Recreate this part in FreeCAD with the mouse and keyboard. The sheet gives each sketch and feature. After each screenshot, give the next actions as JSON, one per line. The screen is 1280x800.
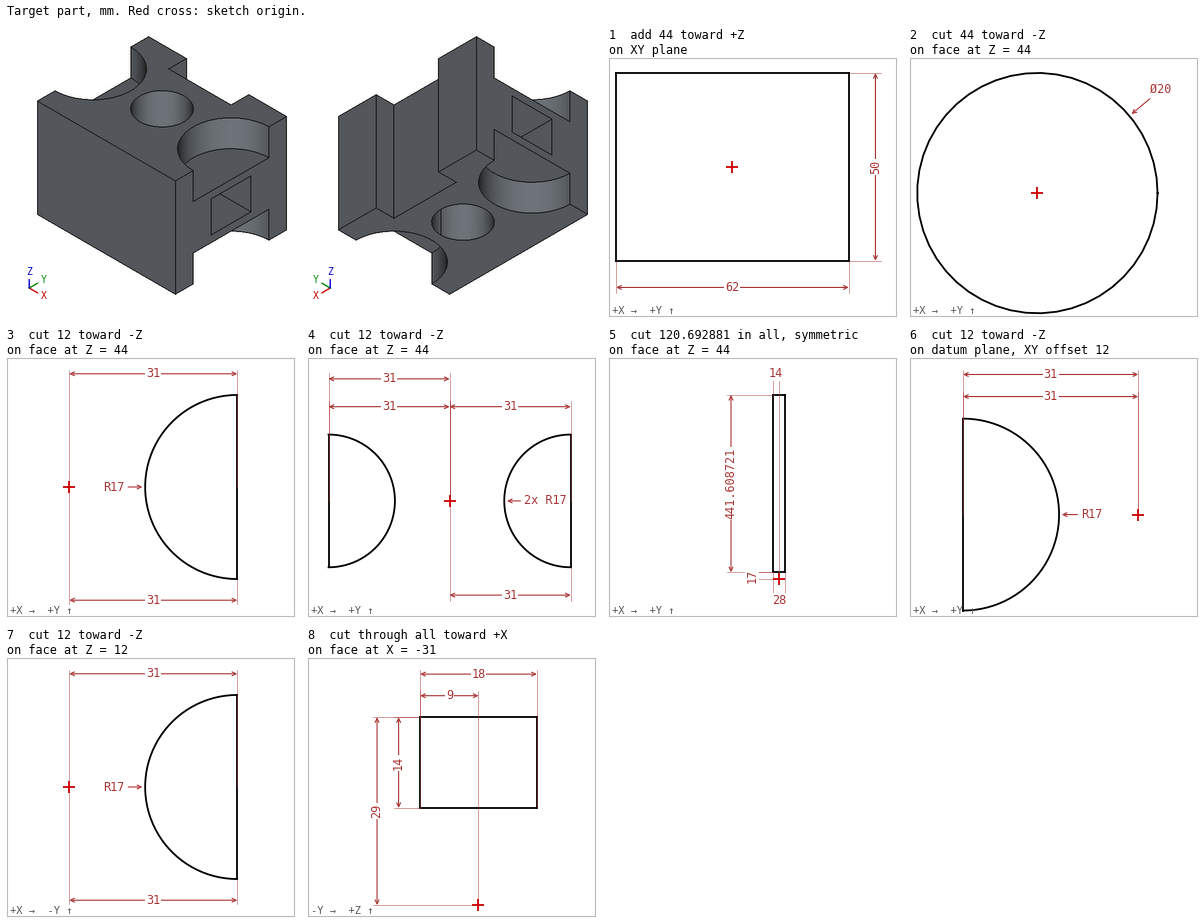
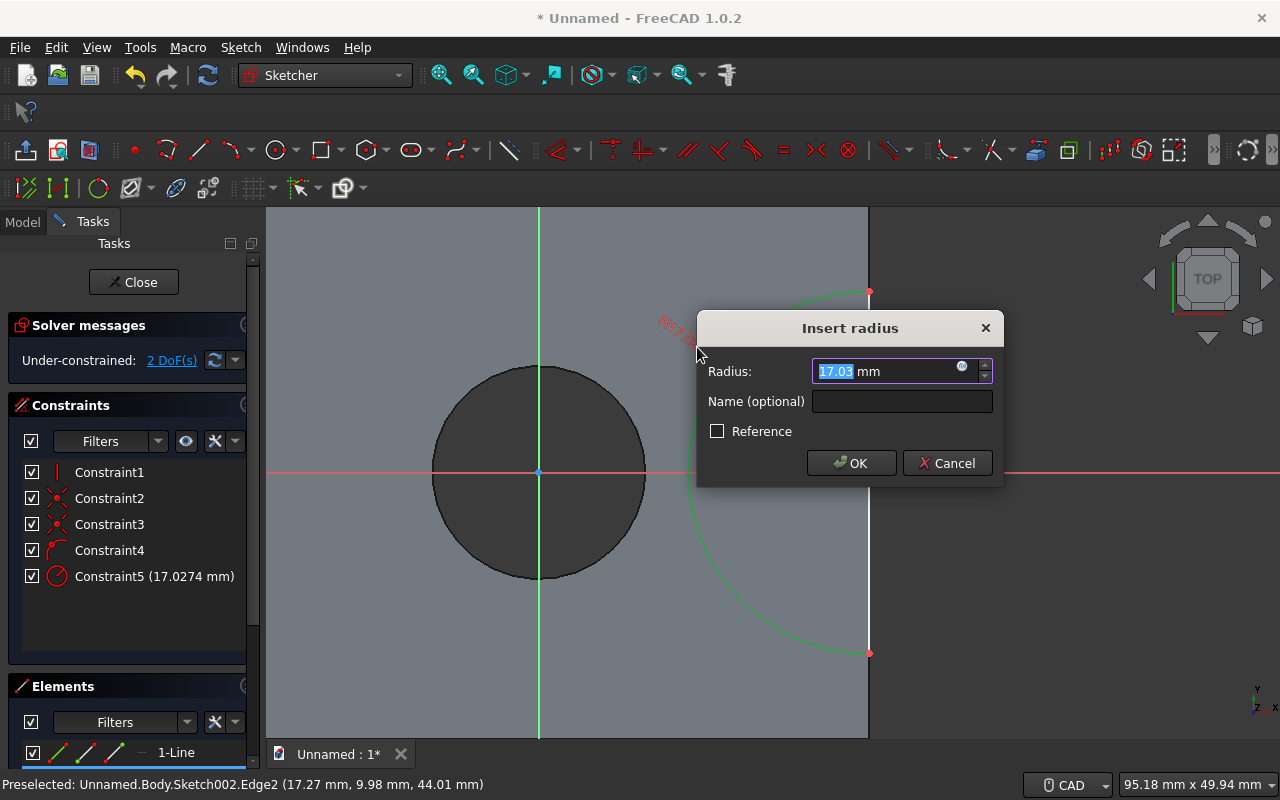
{"action": "type", "text": "17"}
{"action": "key", "text": "Return"}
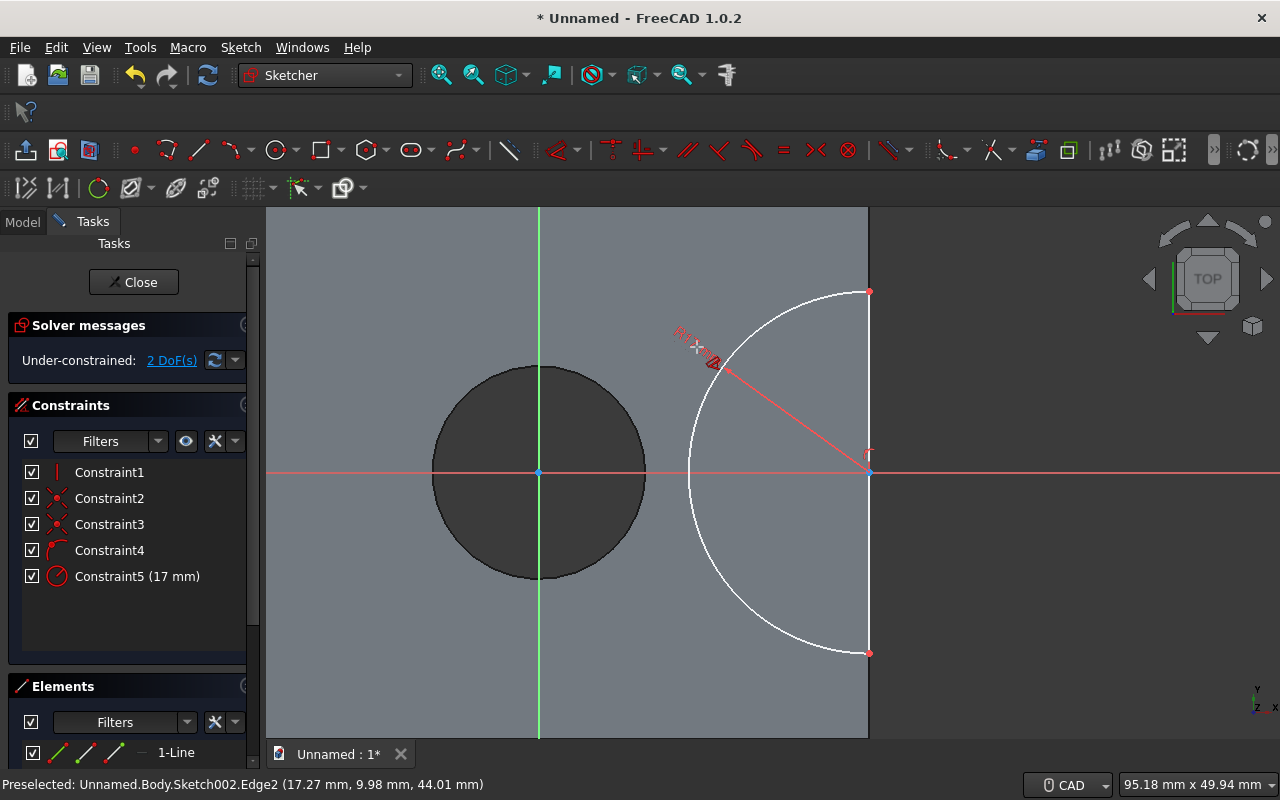
{"action": "left_click", "coordinate": [869, 654]}
{"action": "left_click", "coordinate": [704, 688]}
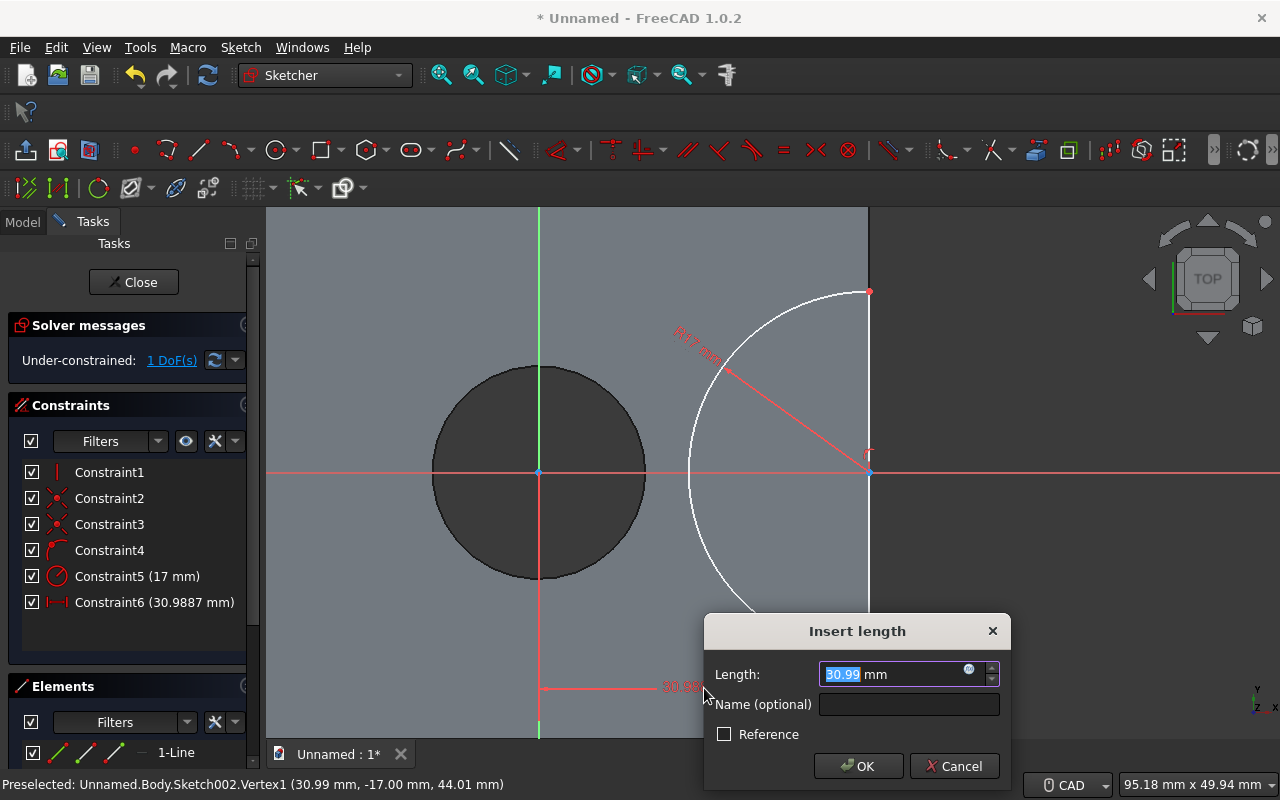
{"action": "type", "text": "31"}
{"action": "key", "text": "Return"}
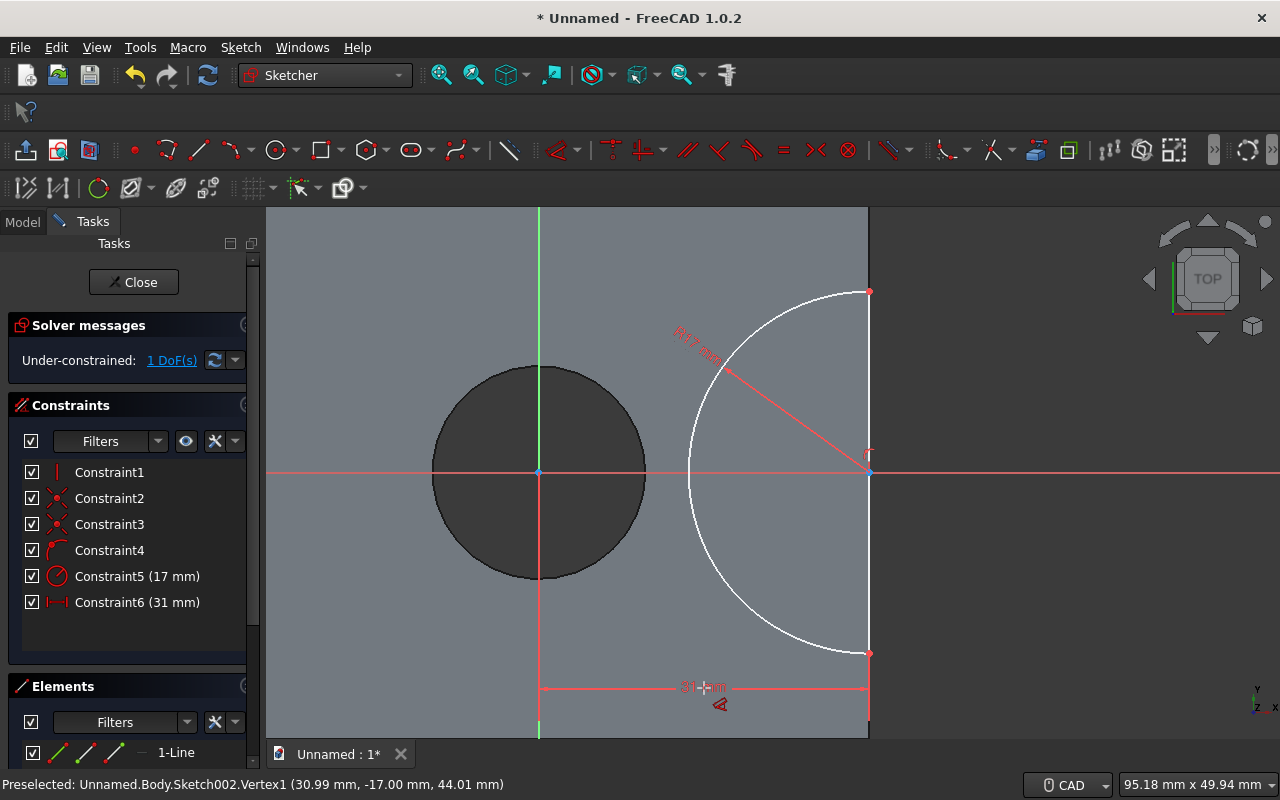
{"action": "left_click", "coordinate": [870, 473]}
{"action": "left_click", "coordinate": [628, 507]}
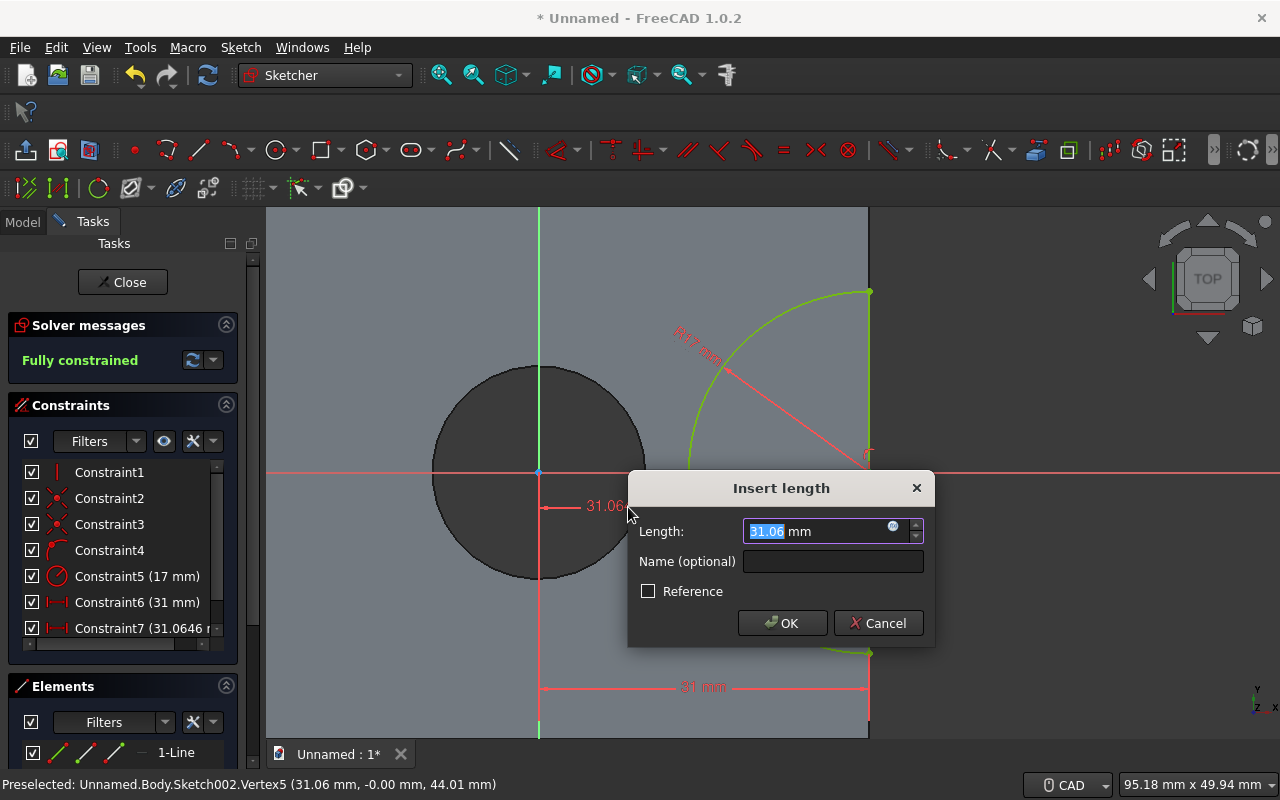
{"action": "type", "text": "31"}
{"action": "key", "text": "Return"}
{"action": "key", "text": "Escape"}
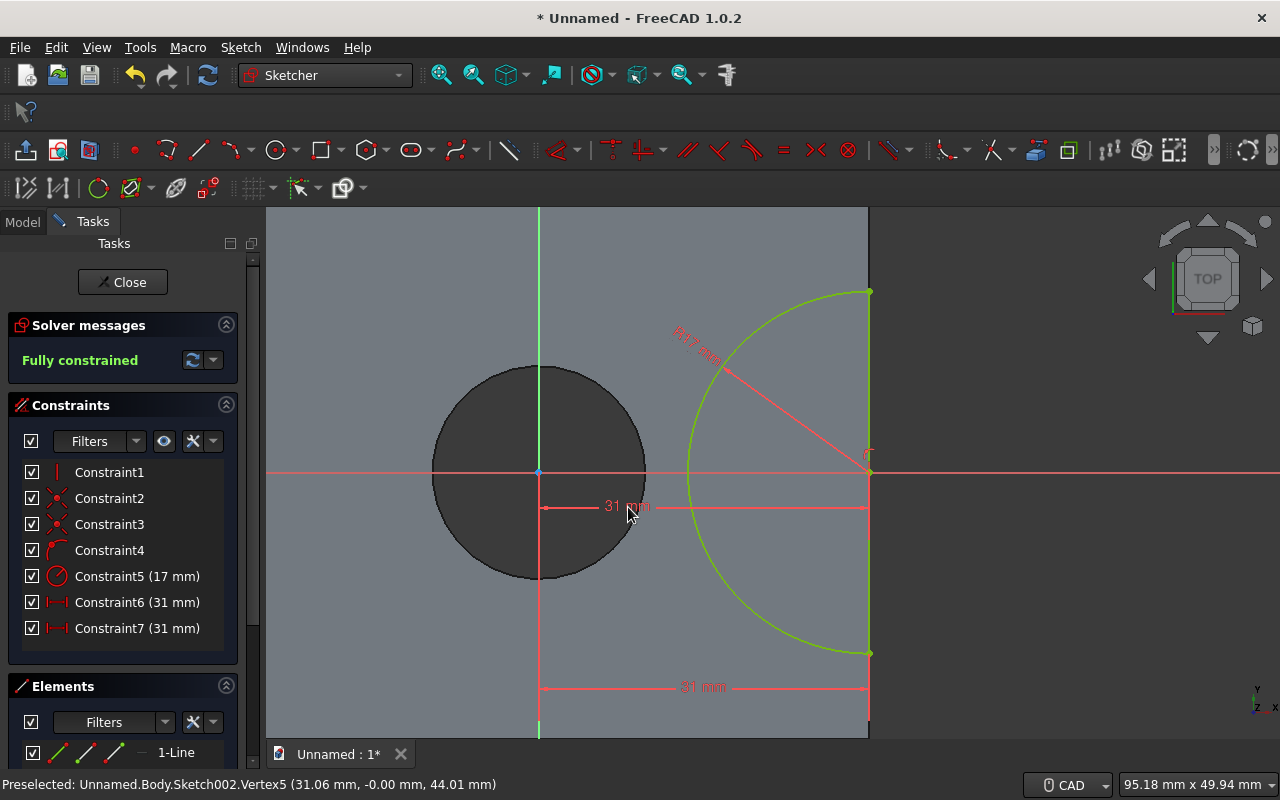
{"action": "left_click", "coordinate": [123, 282]}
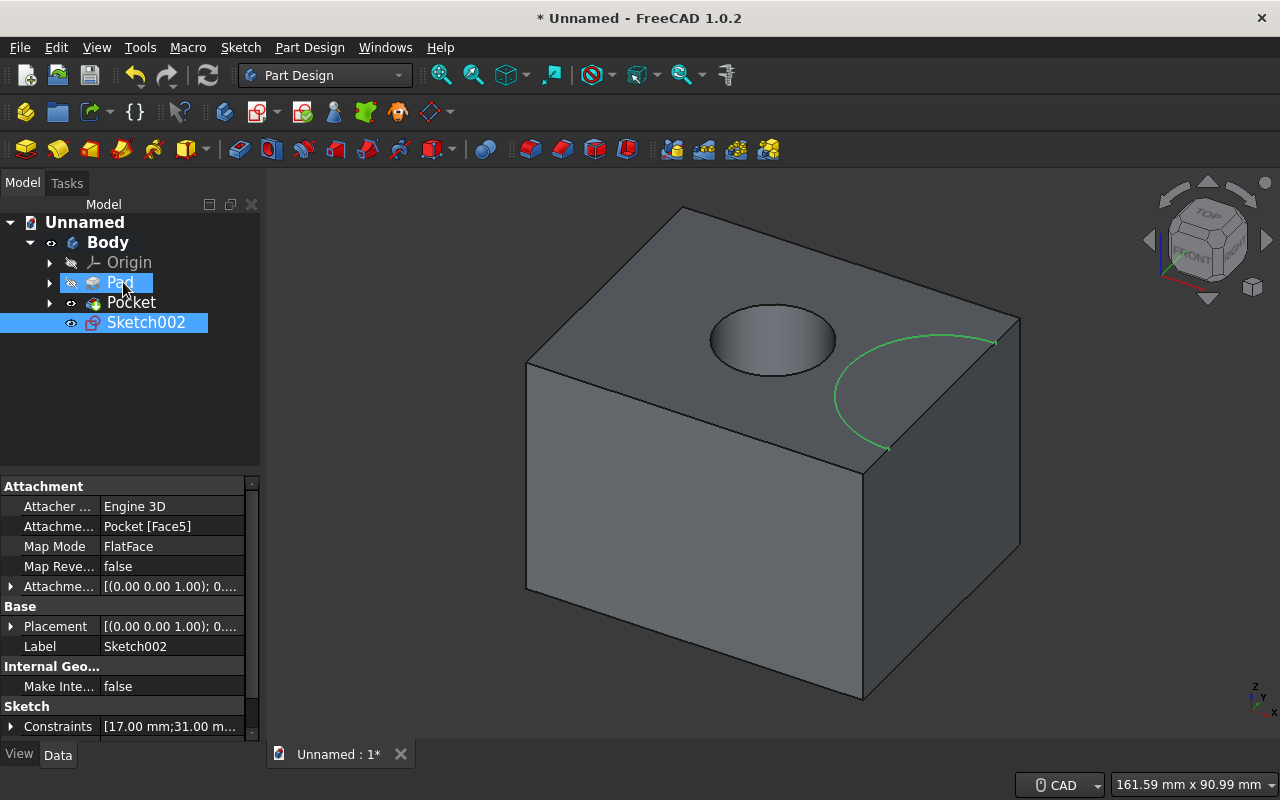
{"action": "left_click", "coordinate": [240, 150]}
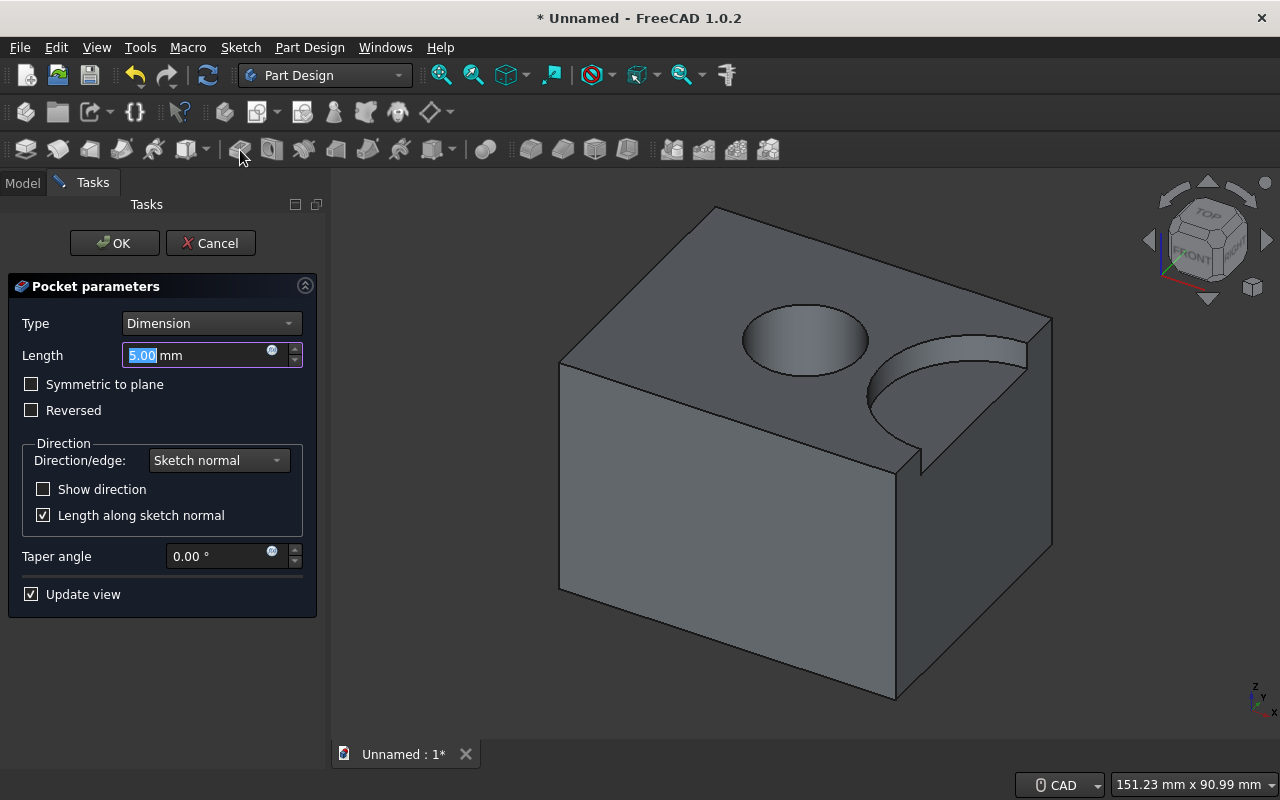
{"action": "type", "text": "12"}
{"action": "key", "text": "Tab"}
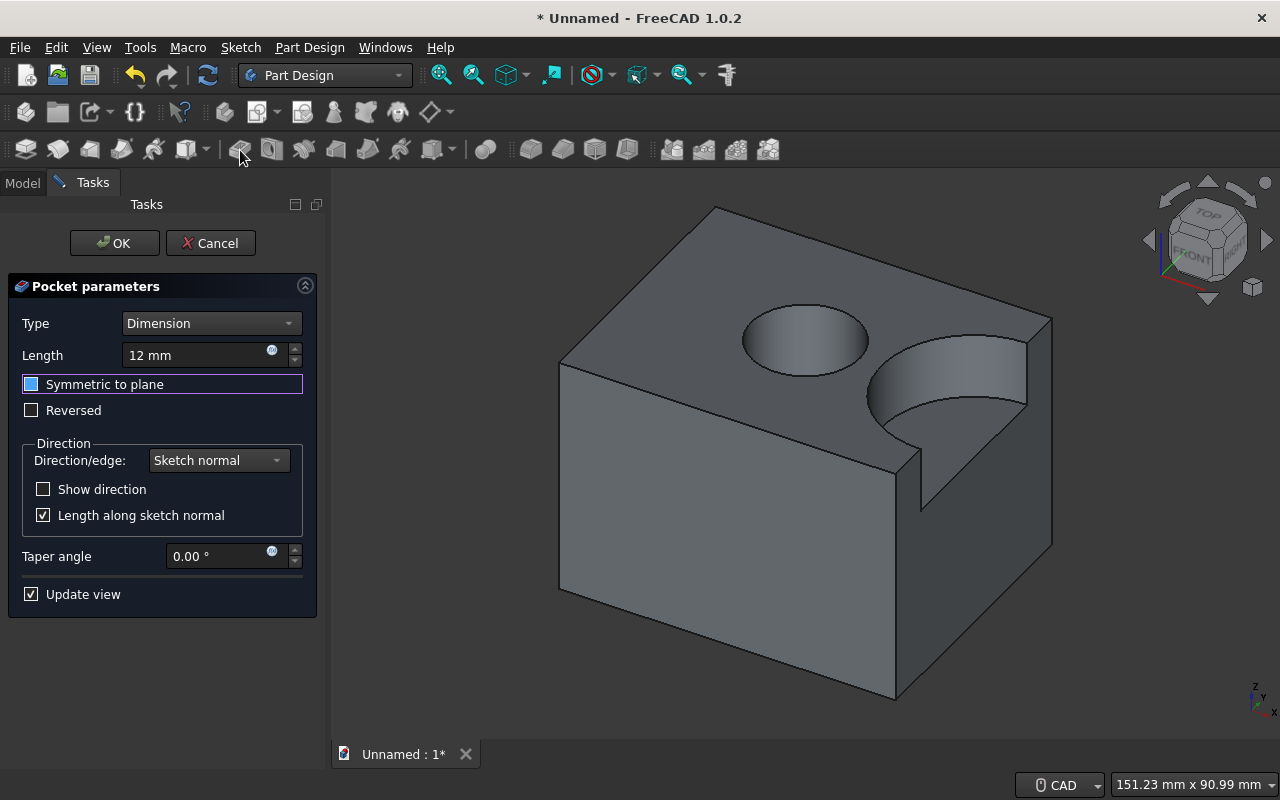
{"action": "left_click", "coordinate": [115, 243]}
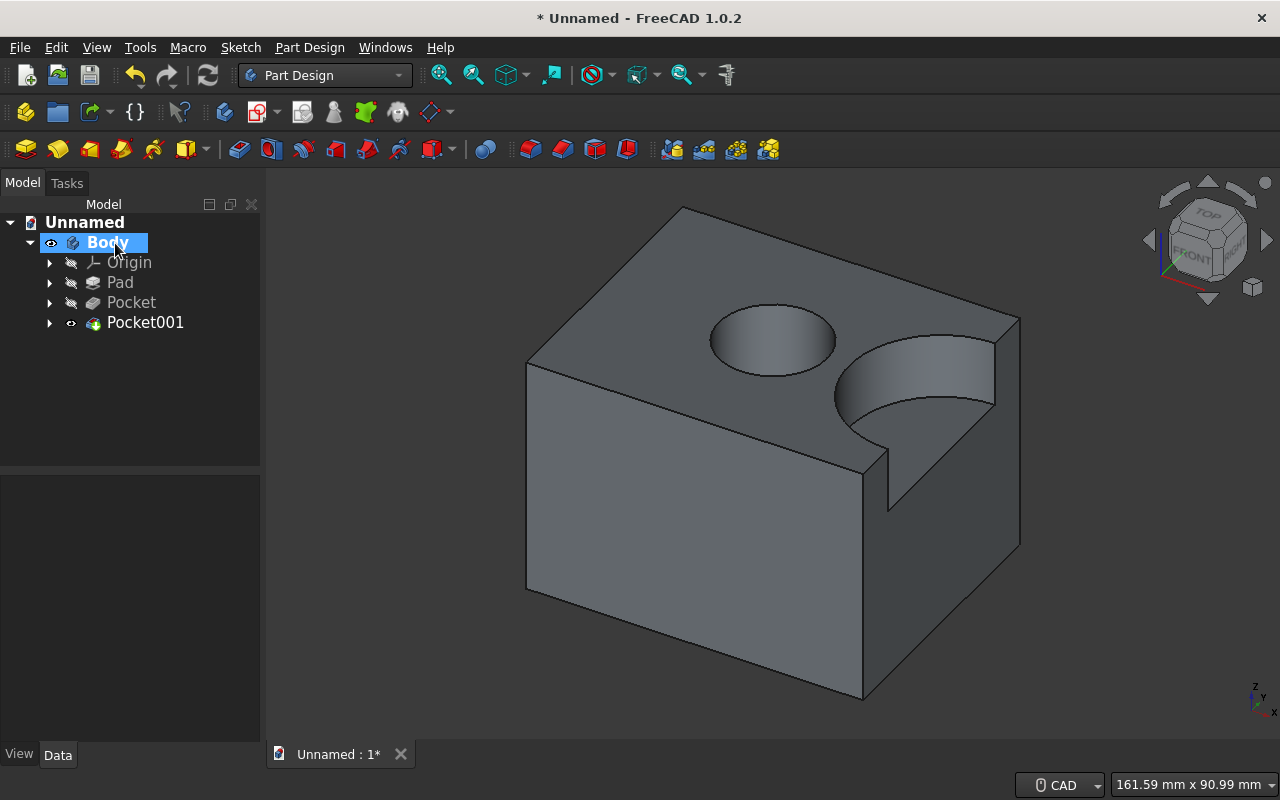
{"action": "left_click", "coordinate": [722, 263]}